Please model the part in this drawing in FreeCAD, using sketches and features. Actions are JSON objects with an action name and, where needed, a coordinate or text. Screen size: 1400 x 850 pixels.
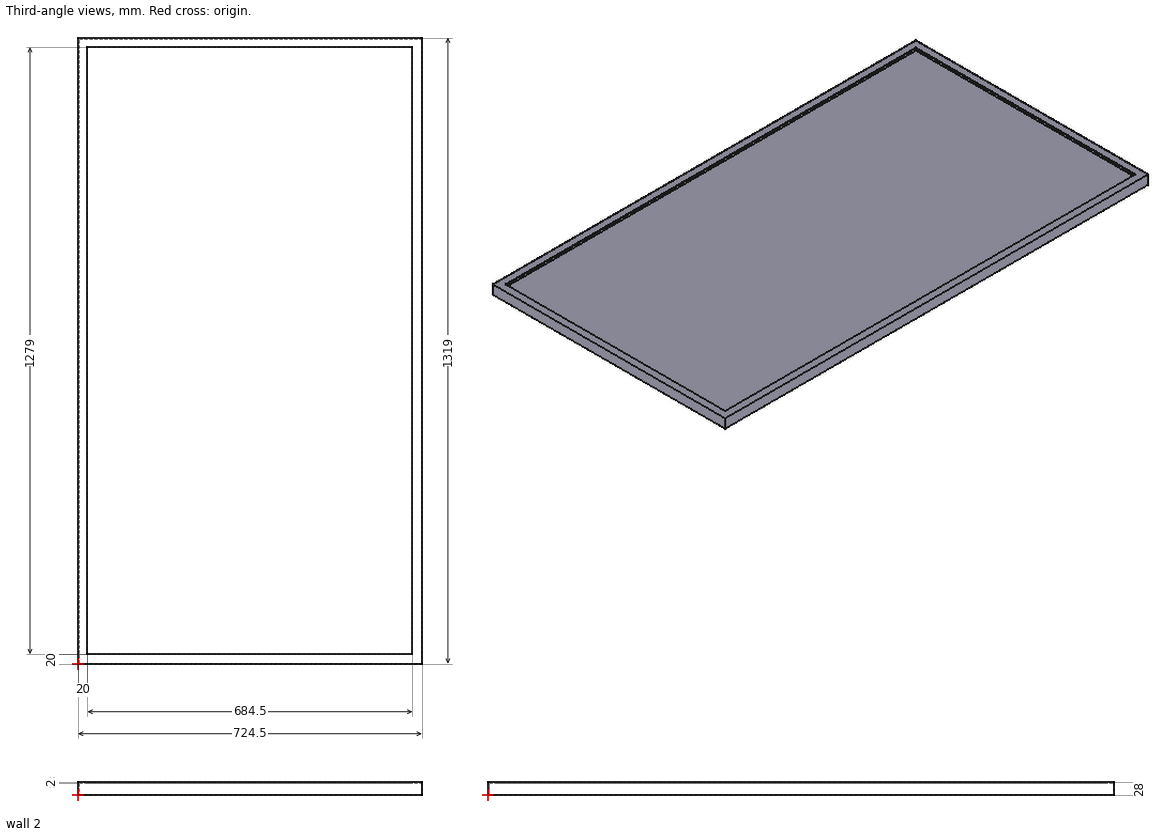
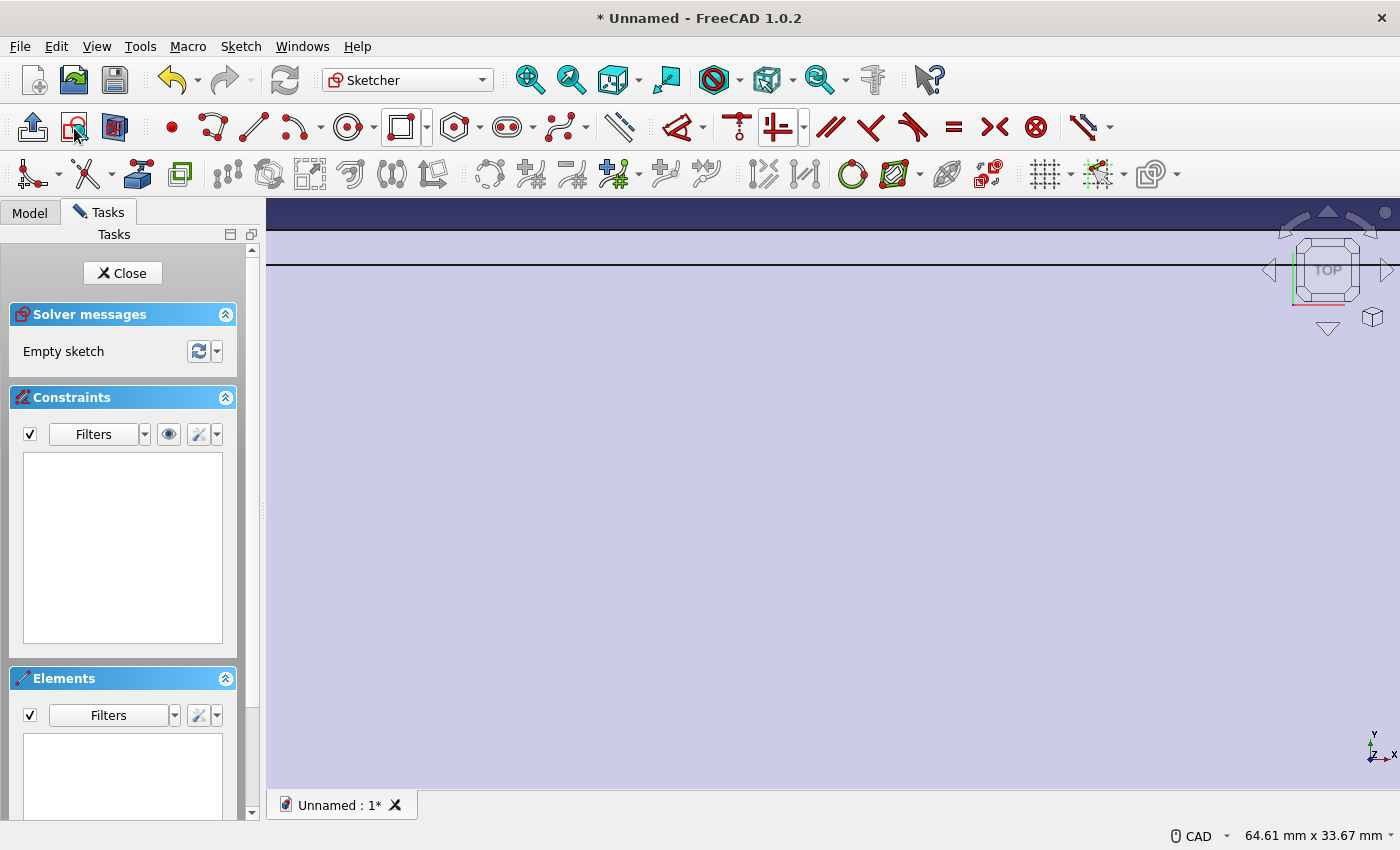
{"action": "scroll", "coordinate": [764, 494], "scroll_direction": "down", "scroll_amount": 15}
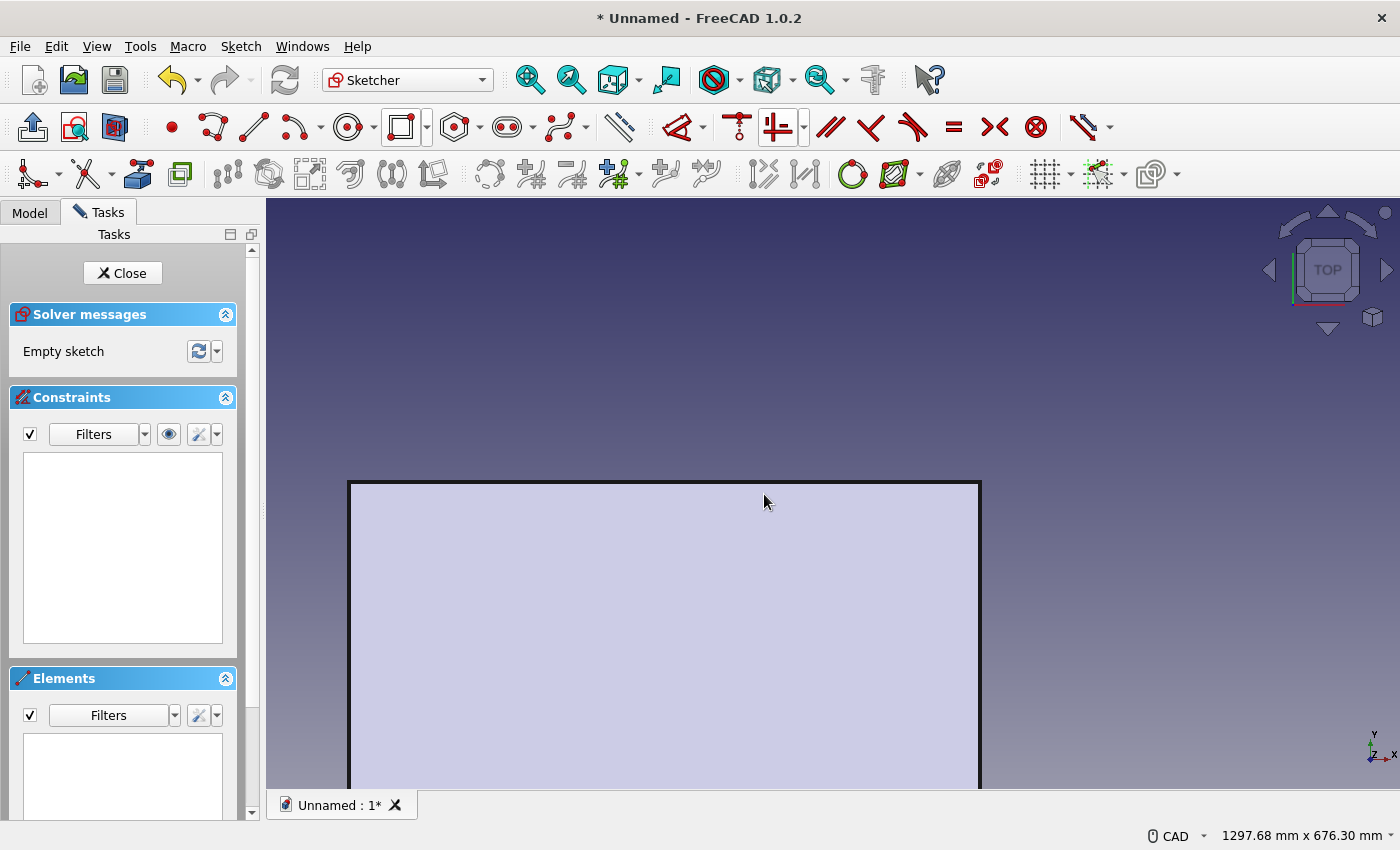
{"action": "scroll", "coordinate": [808, 250], "scroll_direction": "down", "scroll_amount": 6}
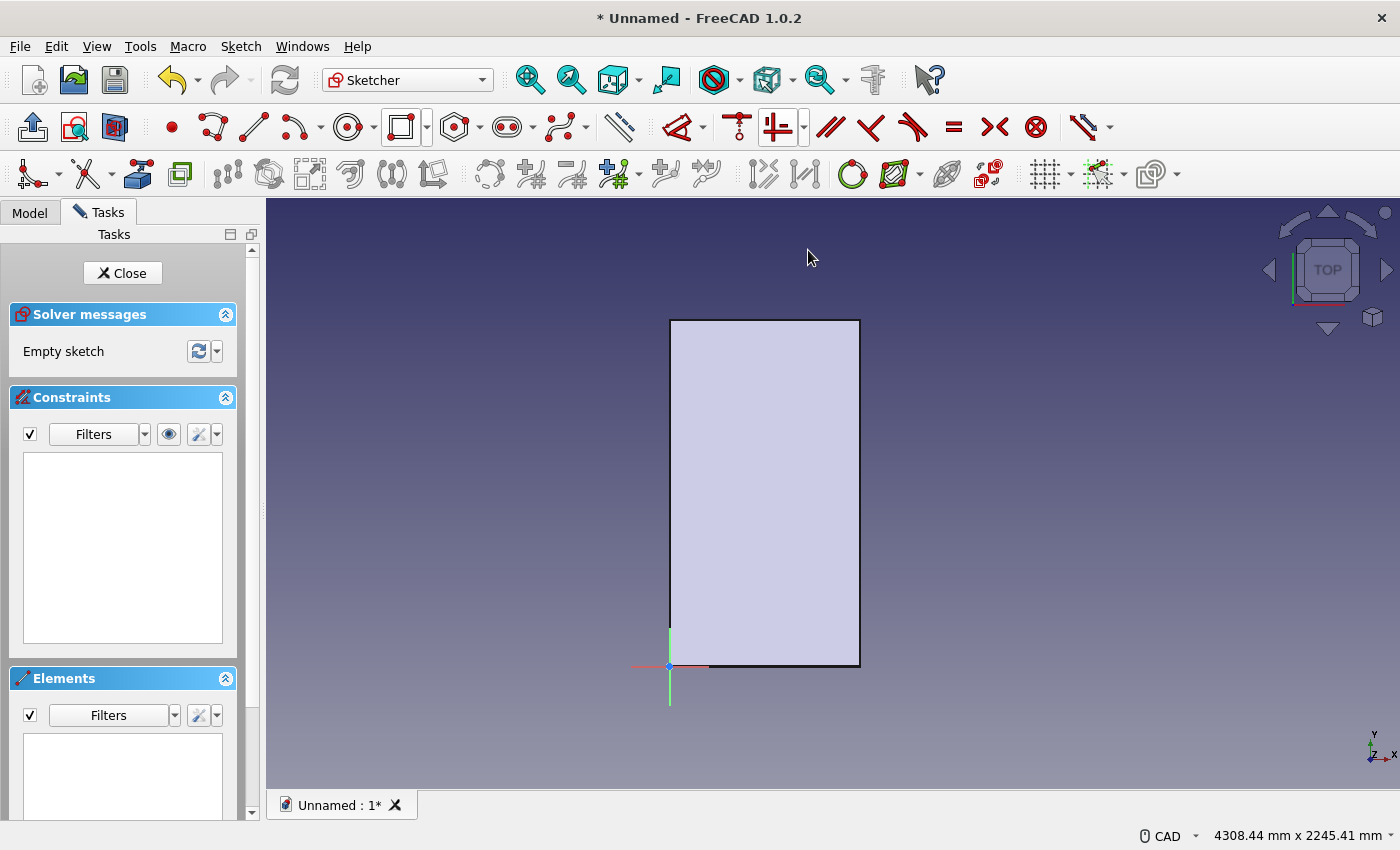
{"action": "left_click", "coordinate": [400, 128]}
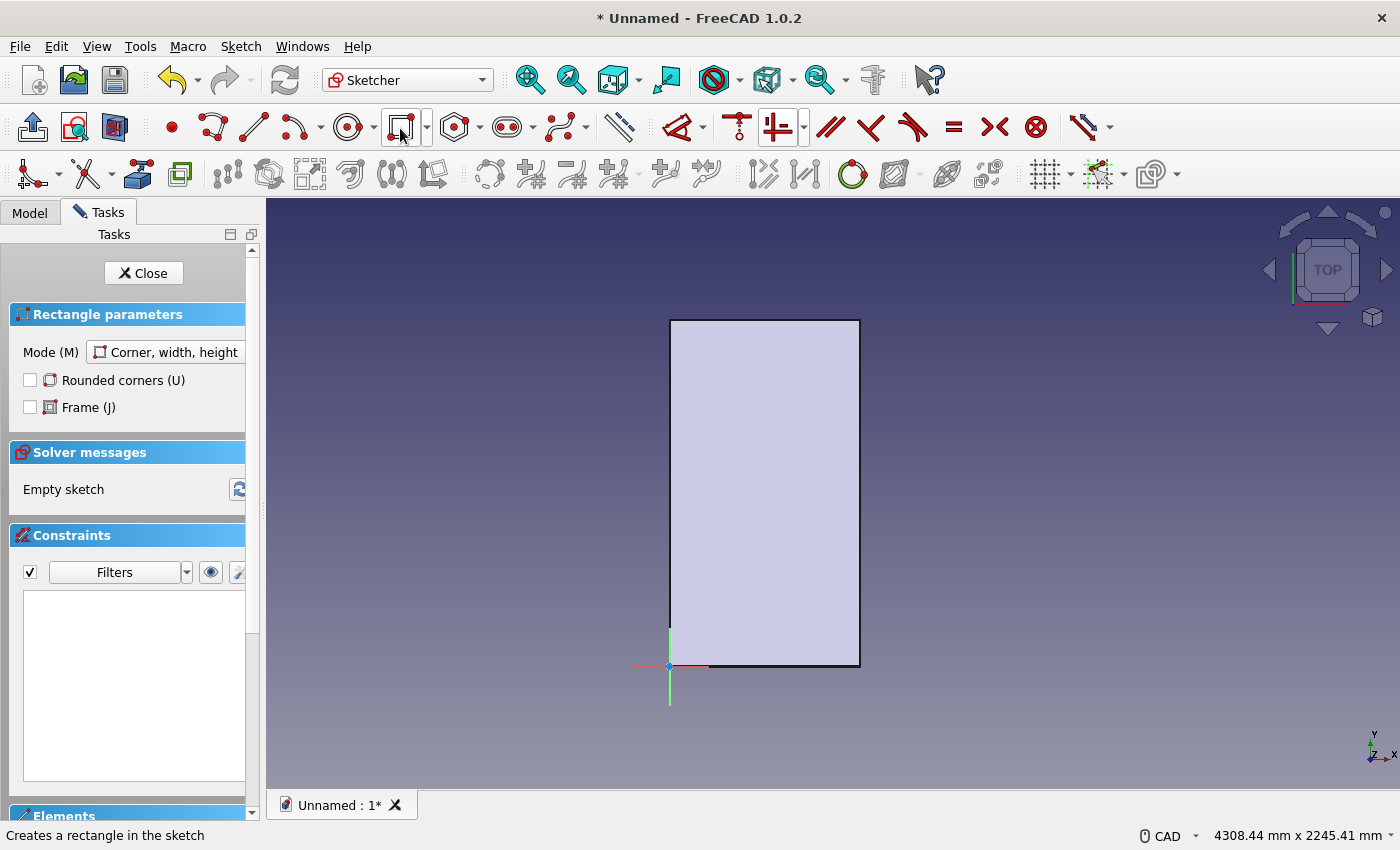
{"action": "left_click", "coordinate": [670, 667]}
{"action": "mouse_move", "coordinate": [860, 320]}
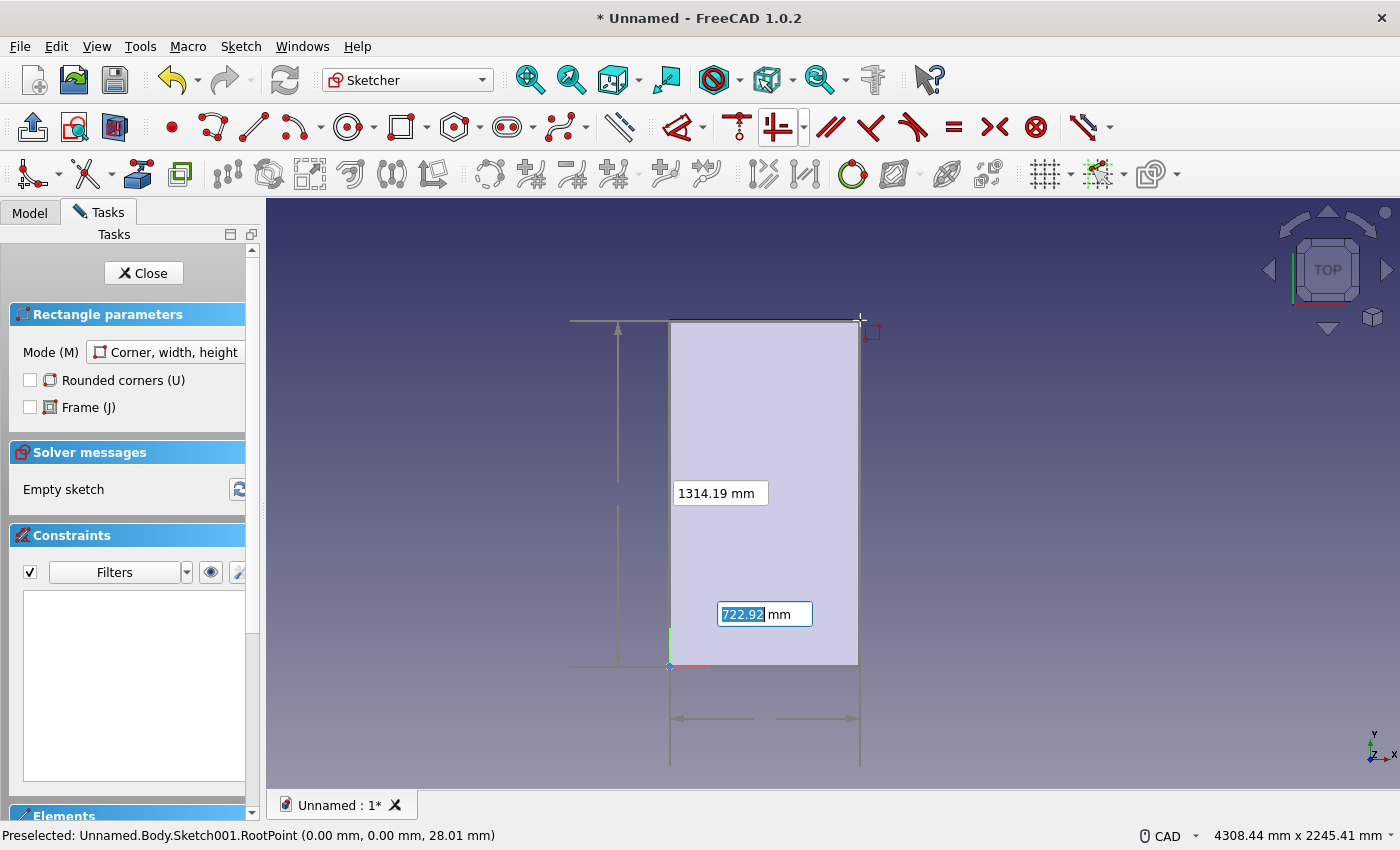
{"action": "type", "text": "724.5"}
{"action": "key", "text": "Tab"}
{"action": "type", "text": "1319"}
{"action": "key", "text": "Return"}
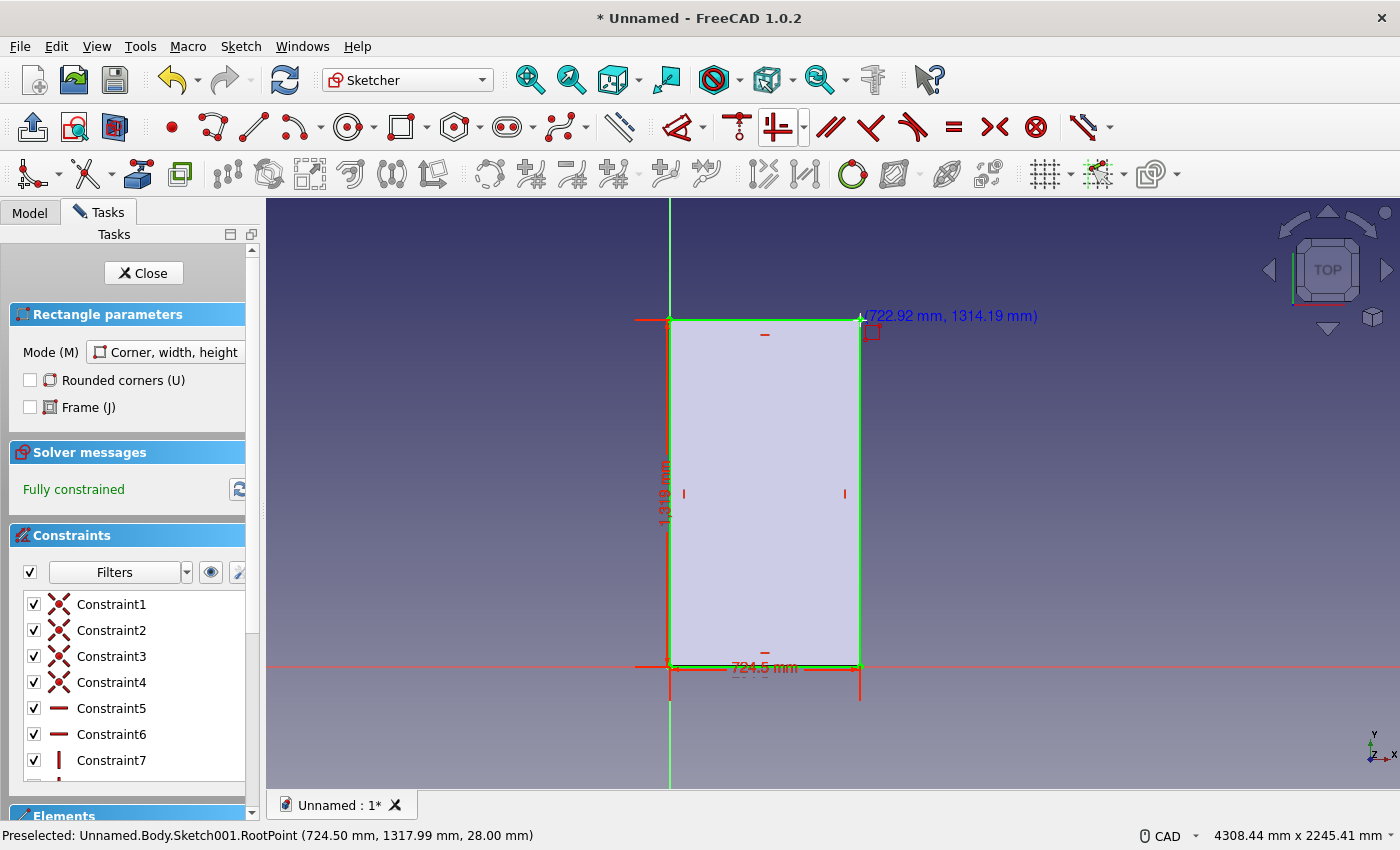
{"action": "scroll", "coordinate": [675, 325], "scroll_direction": "up", "scroll_amount": 6}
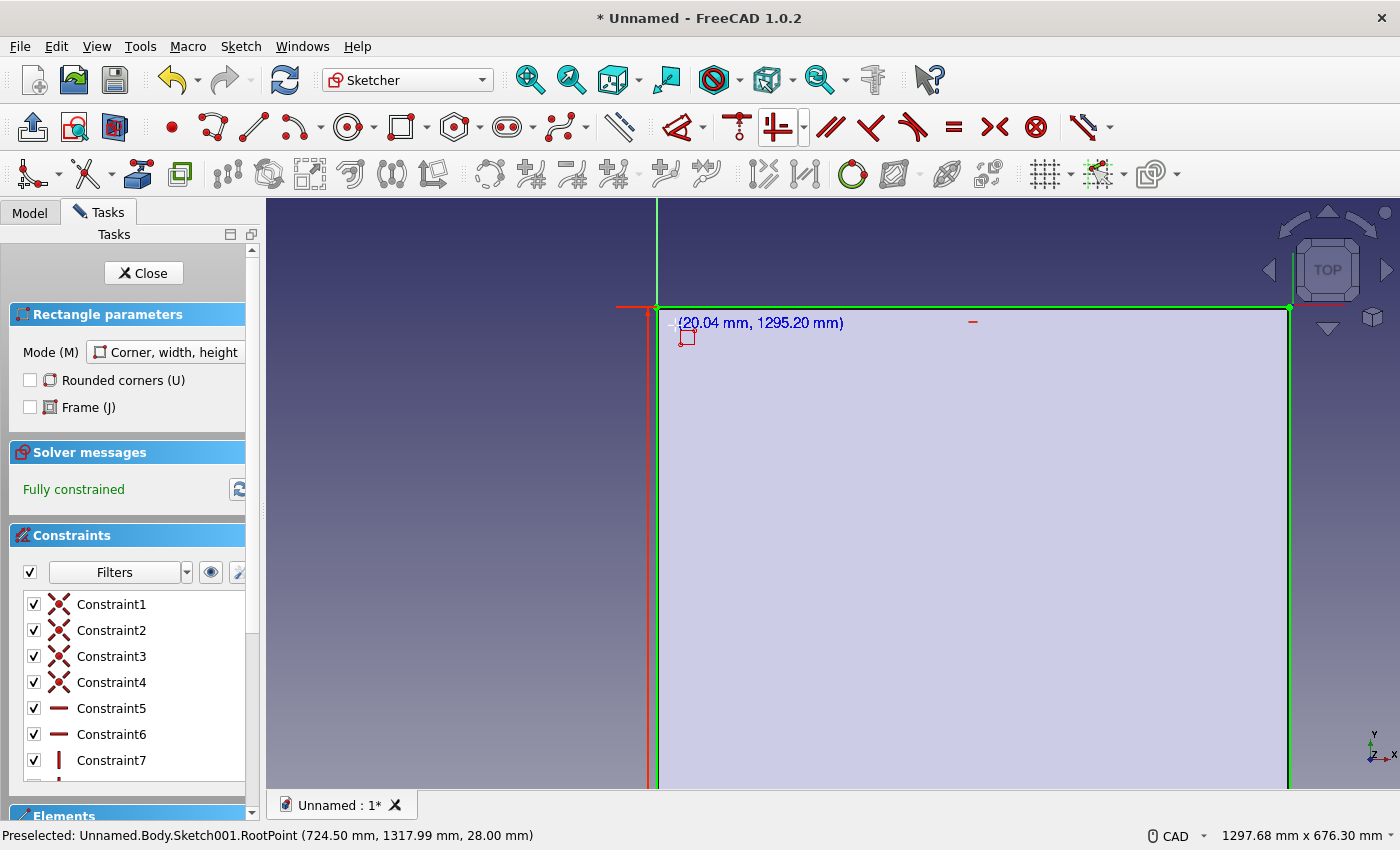
{"action": "left_click", "coordinate": [674, 324]}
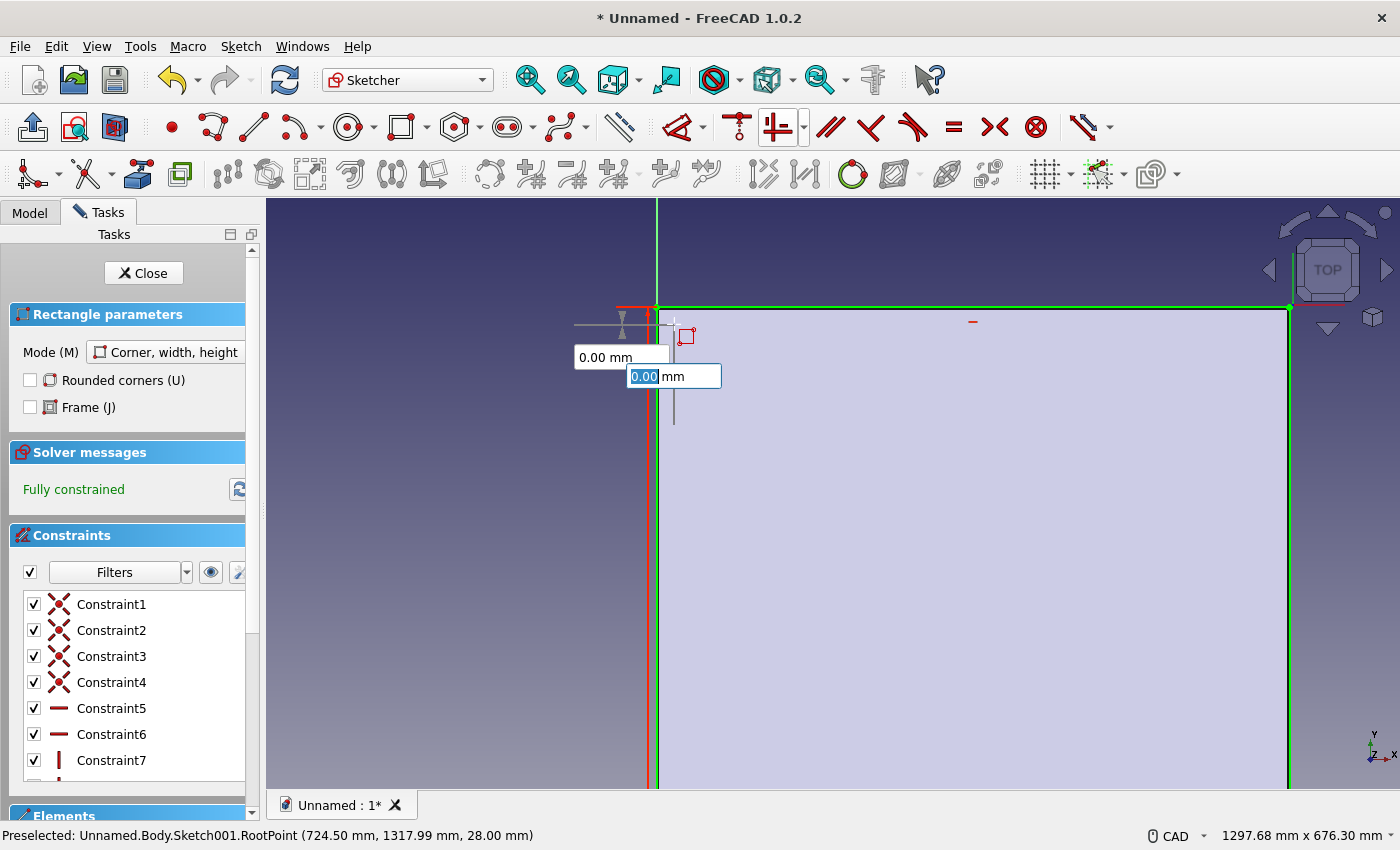
{"action": "scroll", "coordinate": [675, 325], "scroll_direction": "down", "scroll_amount": 6}